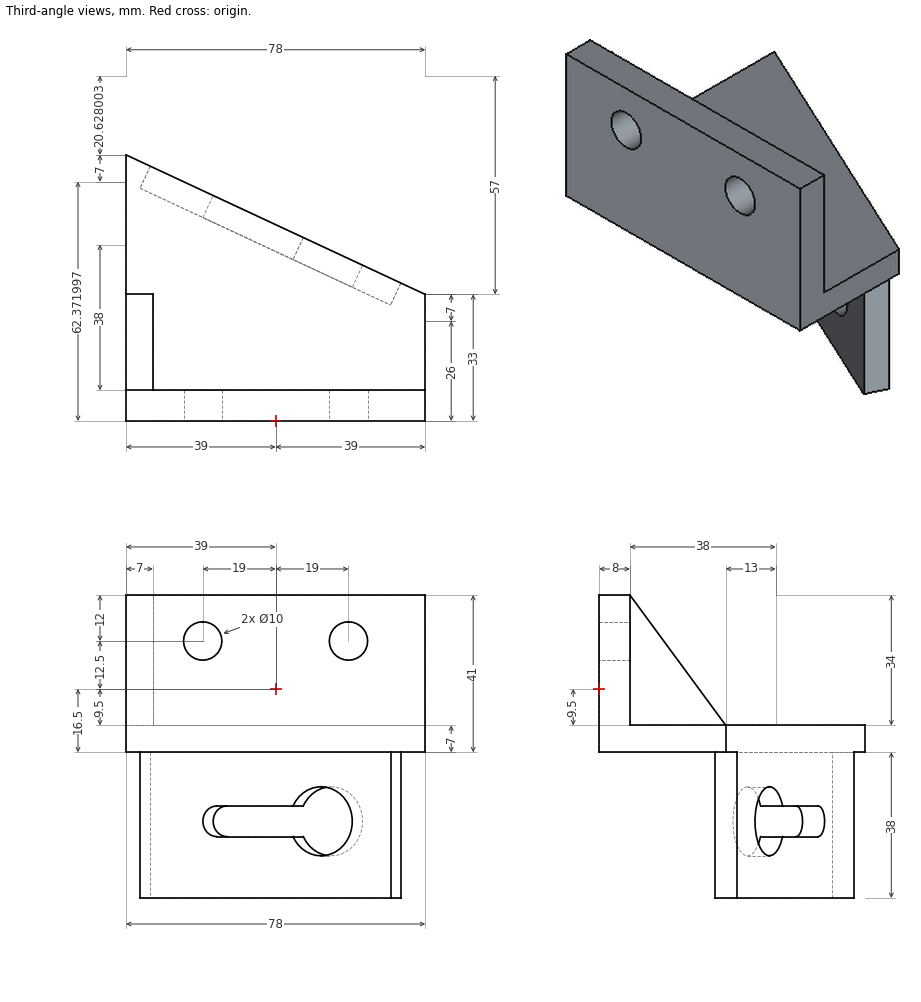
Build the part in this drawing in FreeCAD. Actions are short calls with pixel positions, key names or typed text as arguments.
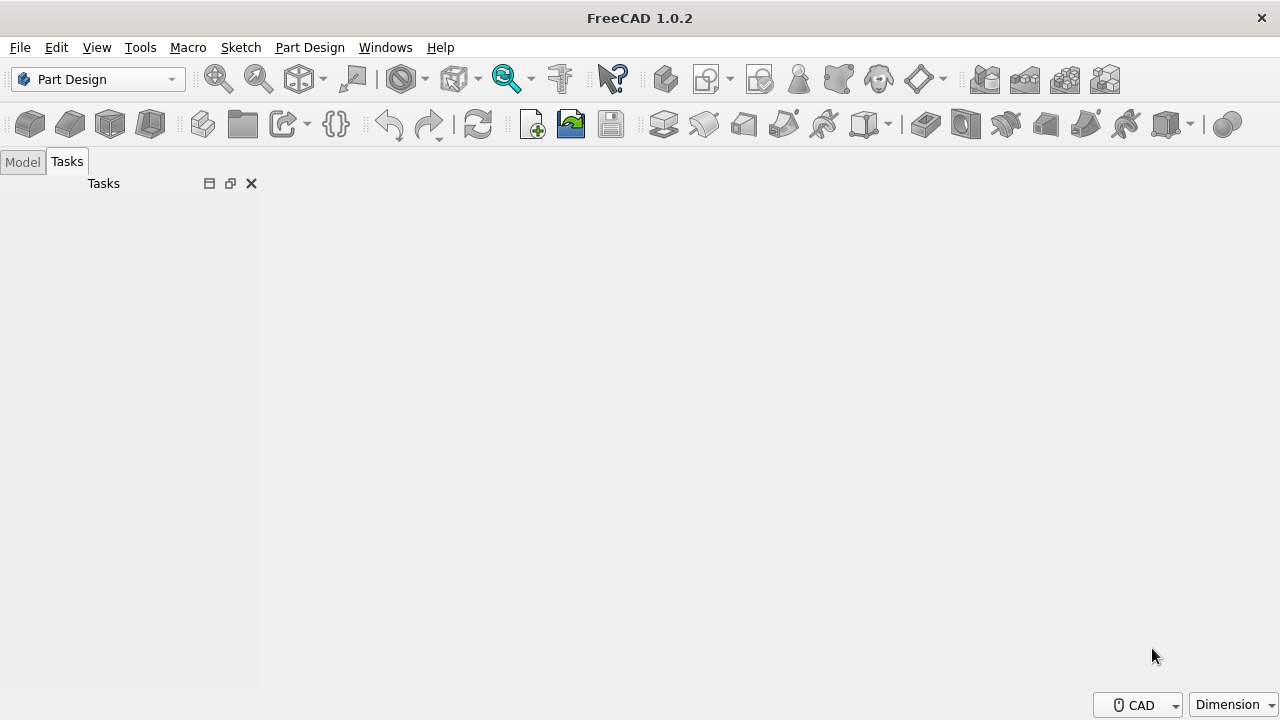
key(ctrl+n)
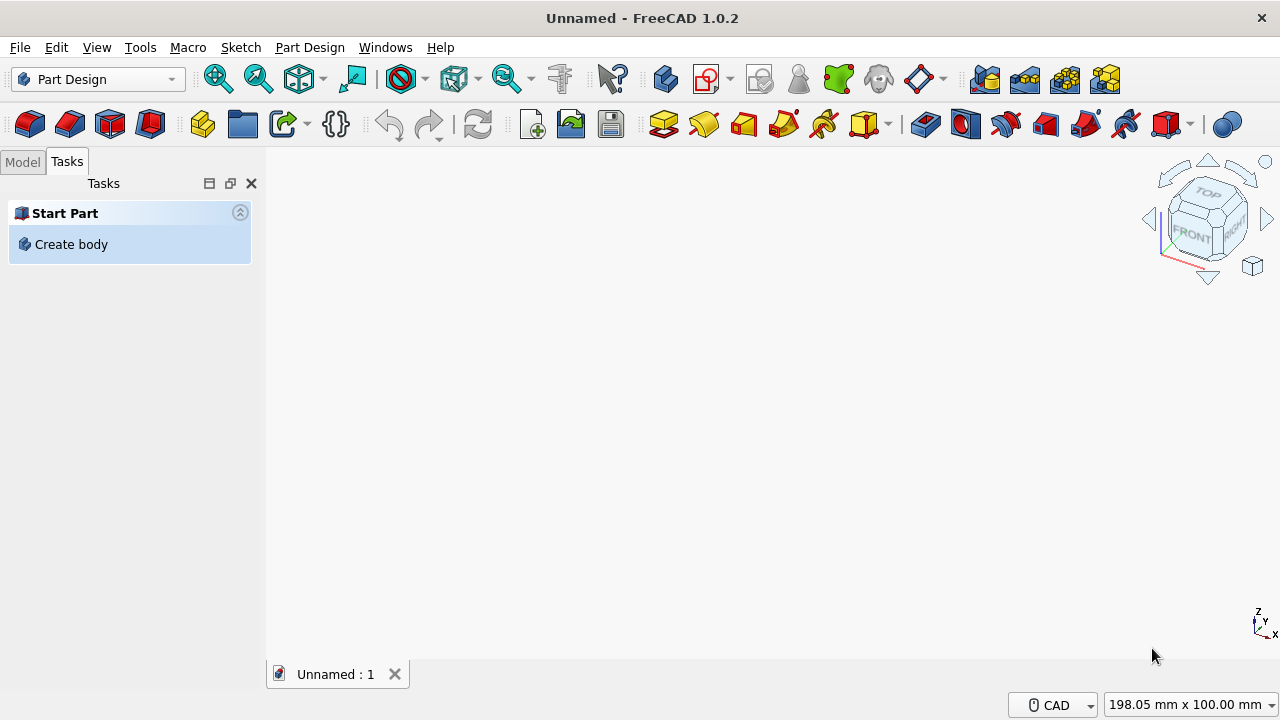
click(706, 80)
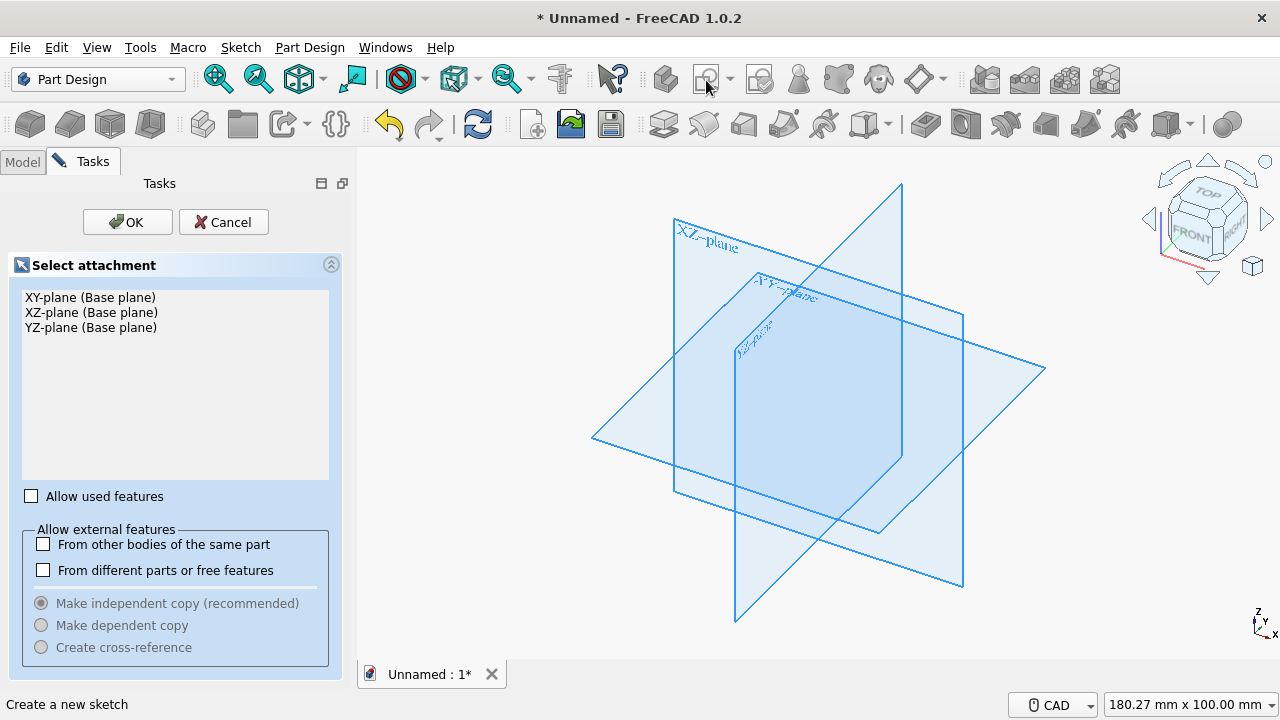
click(82, 312)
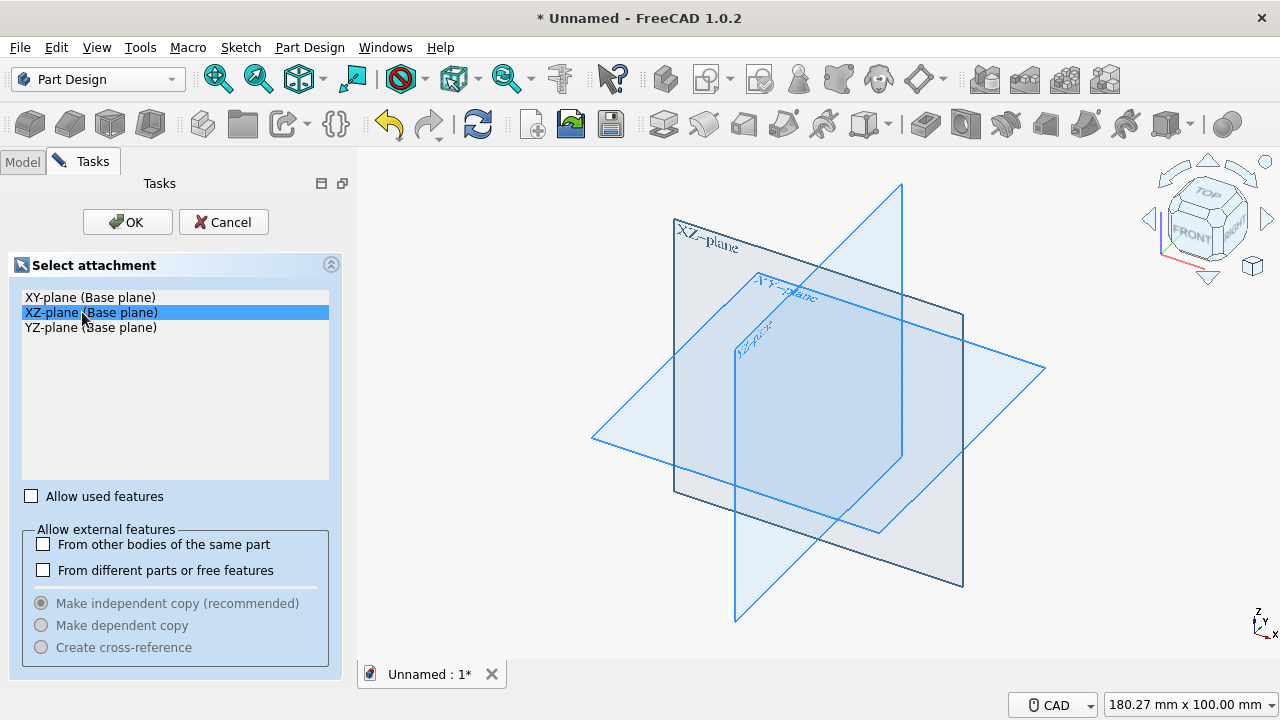
click(128, 222)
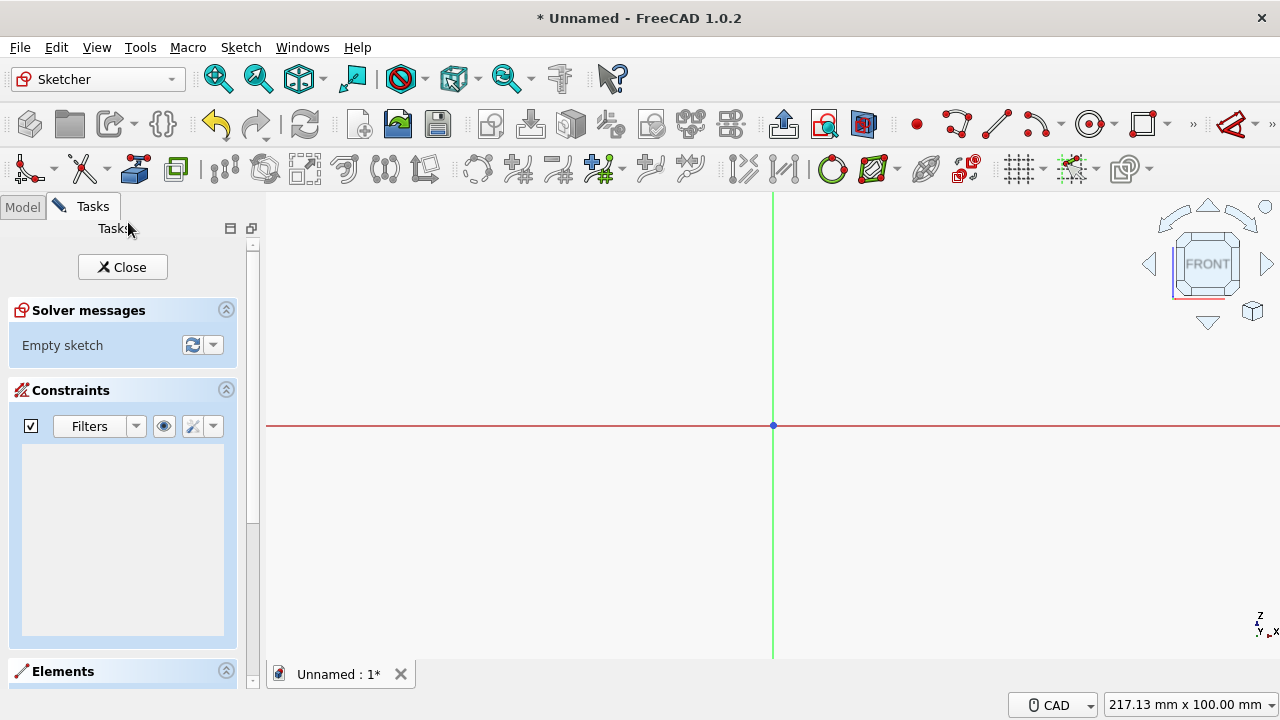
scroll(912, 369, up, 2)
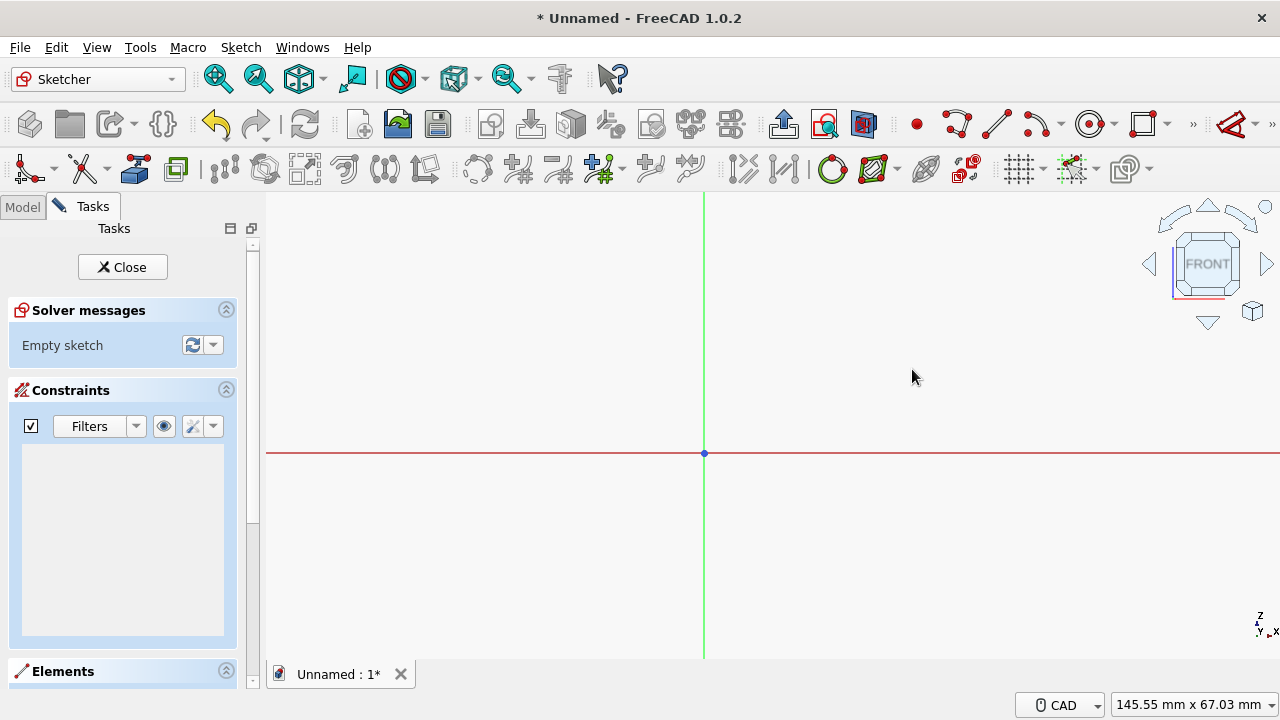
click(1144, 124)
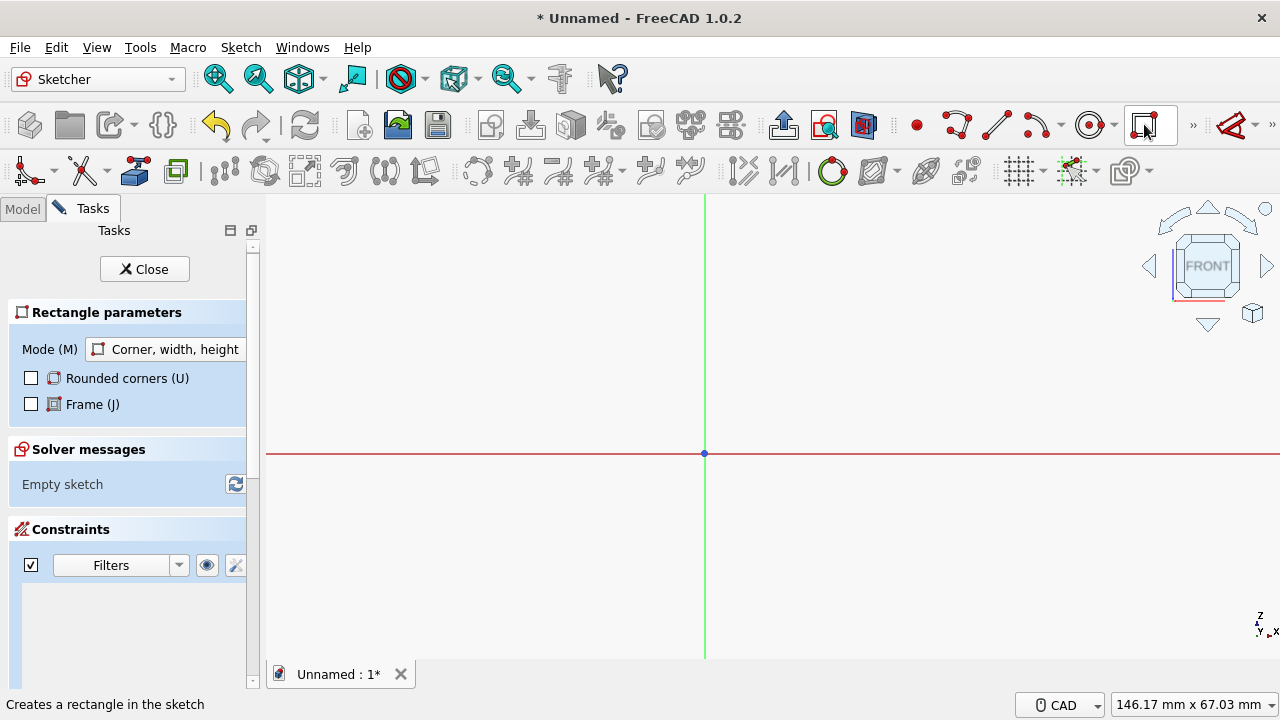
click(434, 284)
move(975, 568)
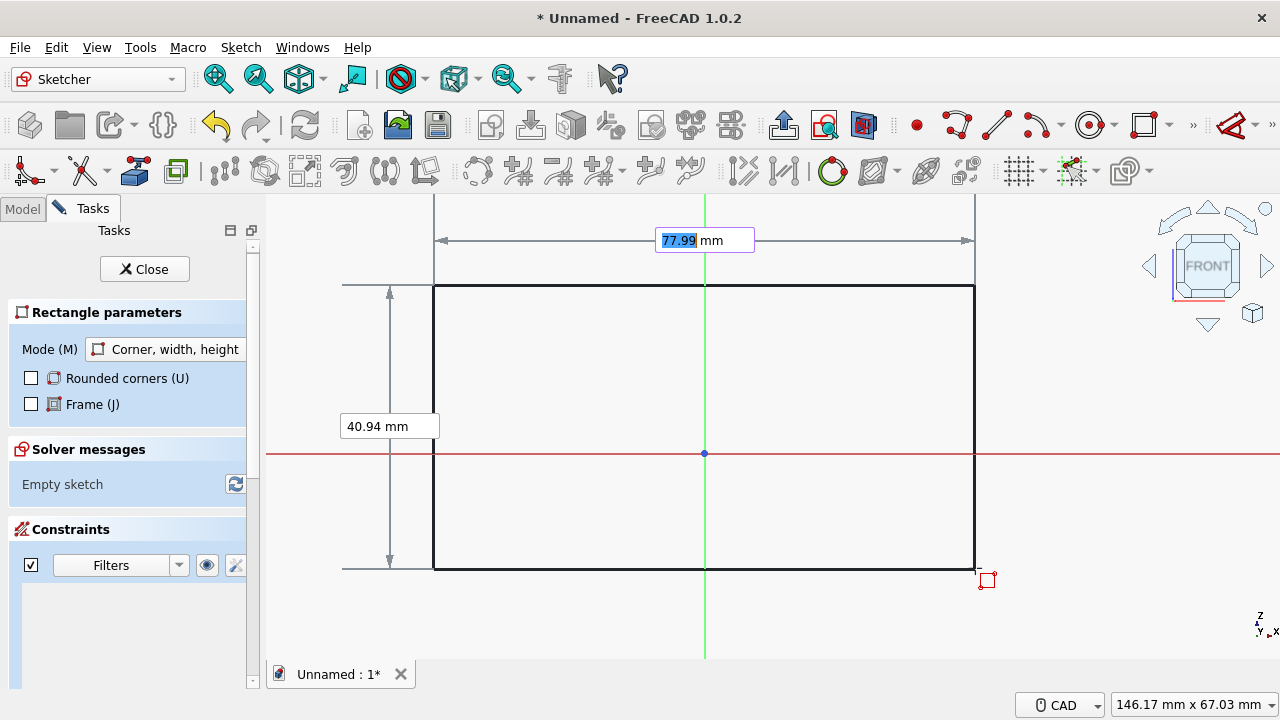
text(78)
key(Tab)
text(41)
key(Return)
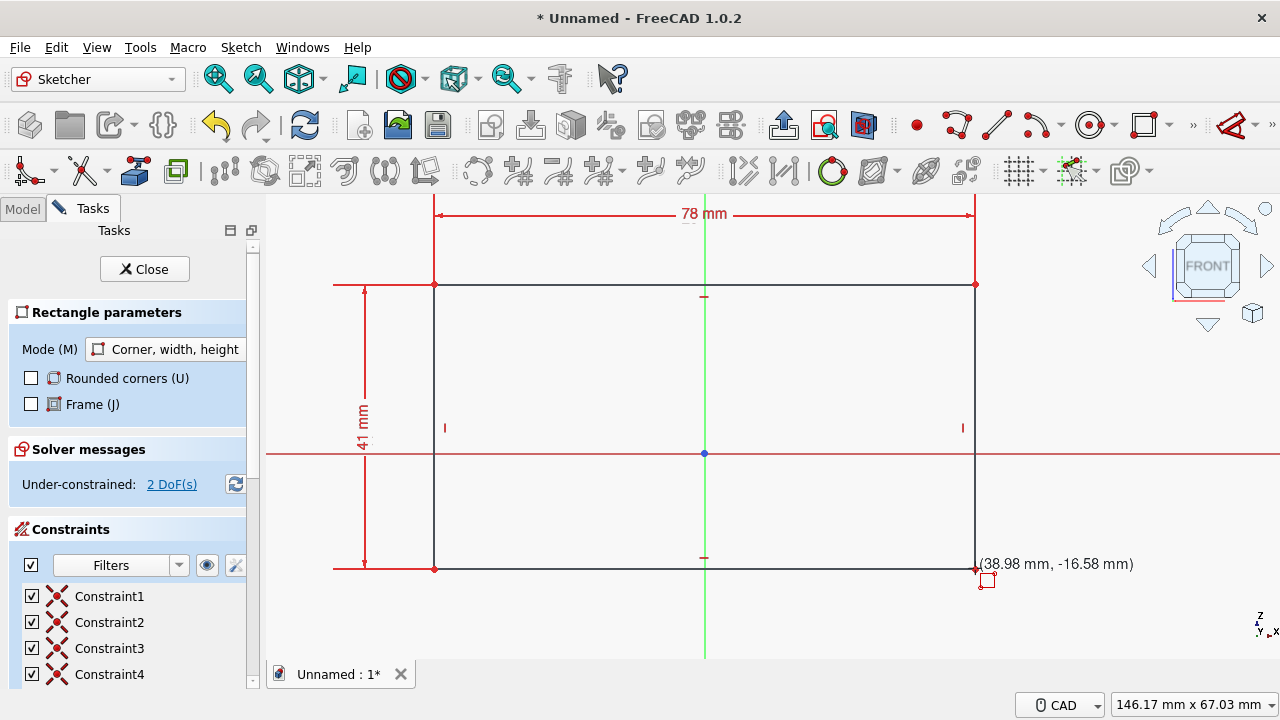
click(1090, 126)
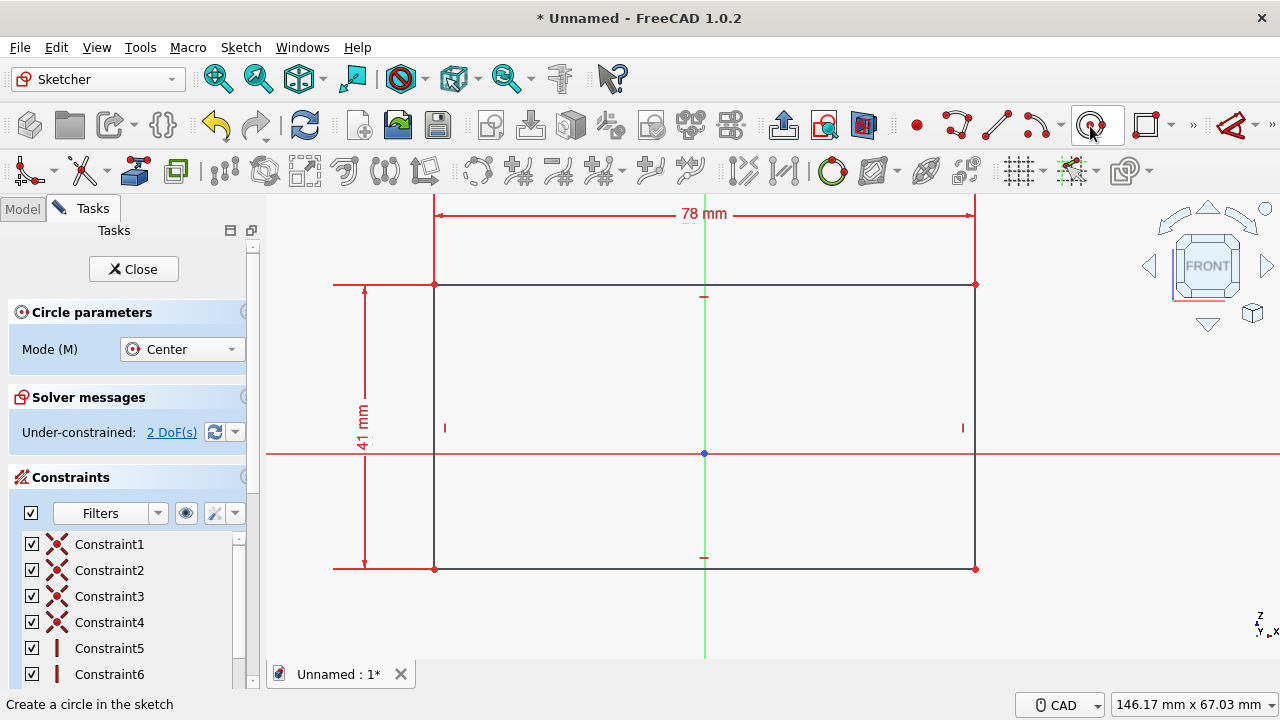
click(573, 367)
move(597, 343)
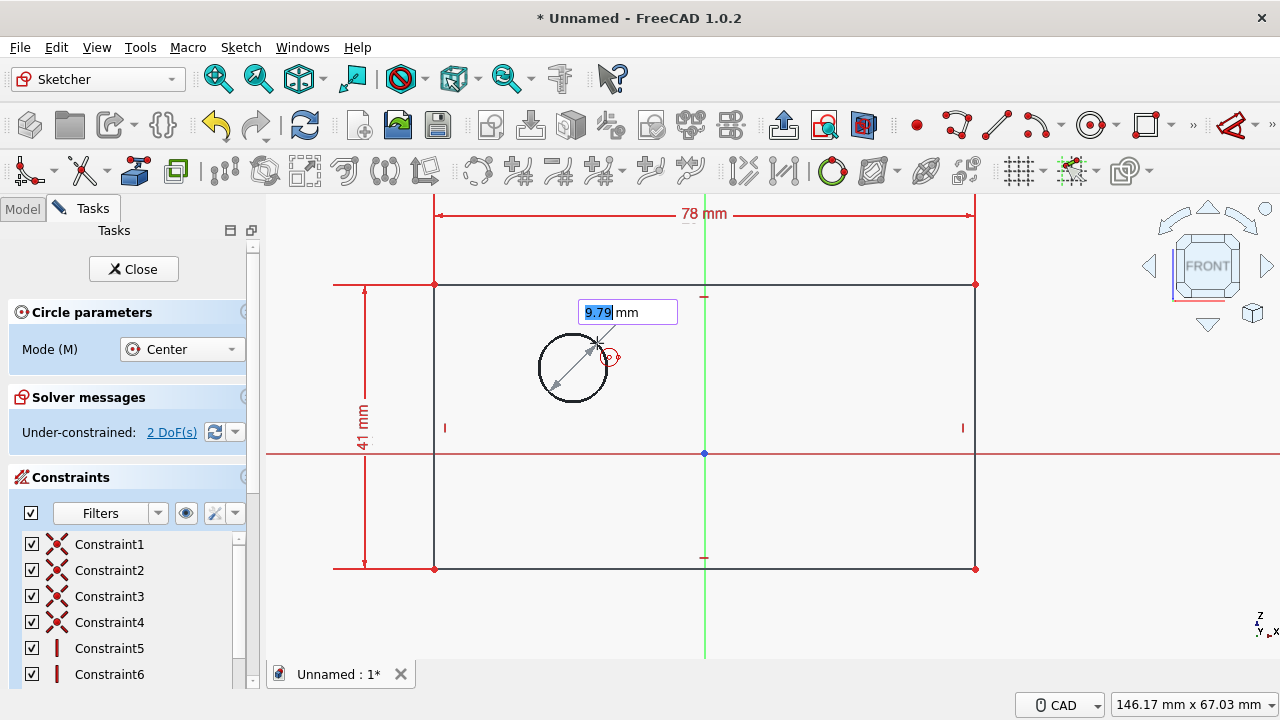
text(10)
key(Return)